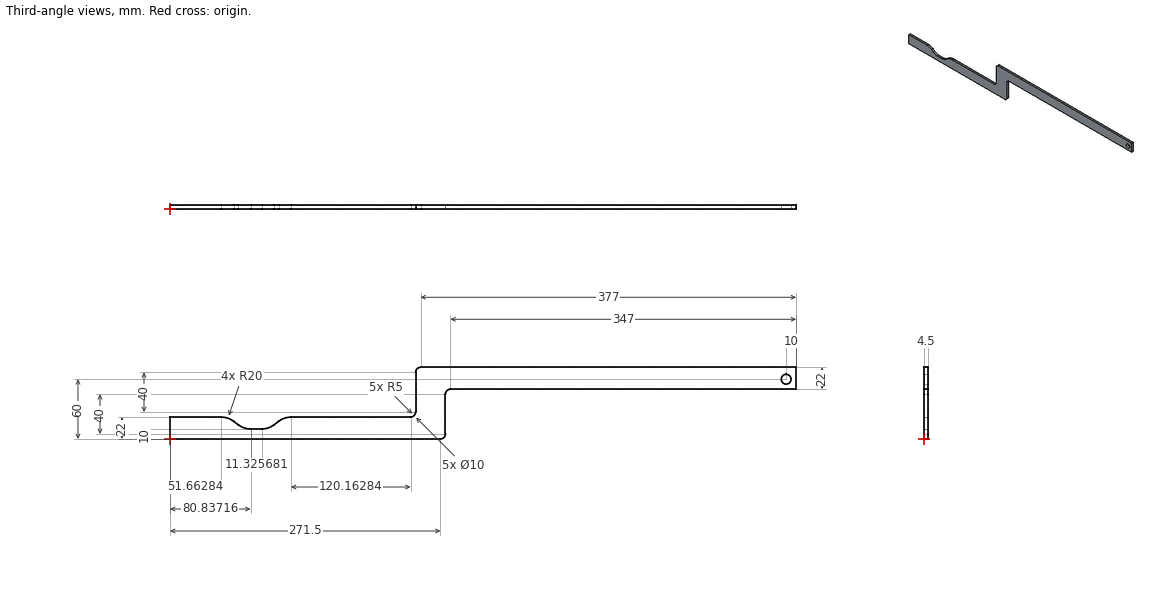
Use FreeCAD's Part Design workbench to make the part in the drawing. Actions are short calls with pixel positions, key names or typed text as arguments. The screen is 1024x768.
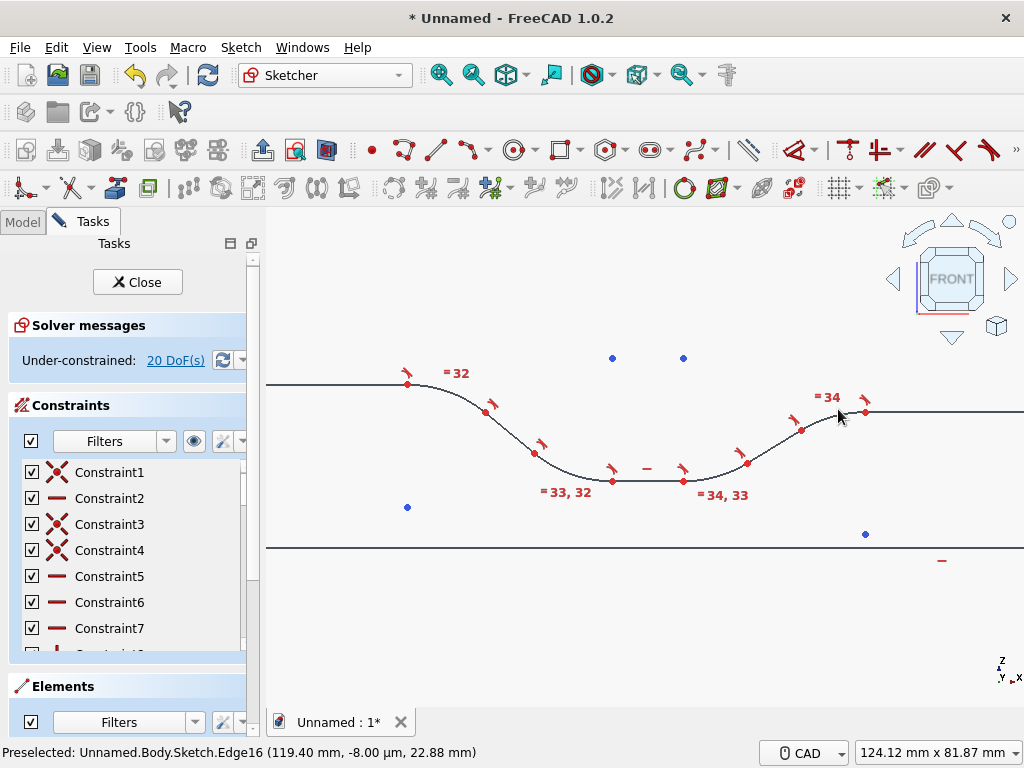
scroll(395, 473, down, 11)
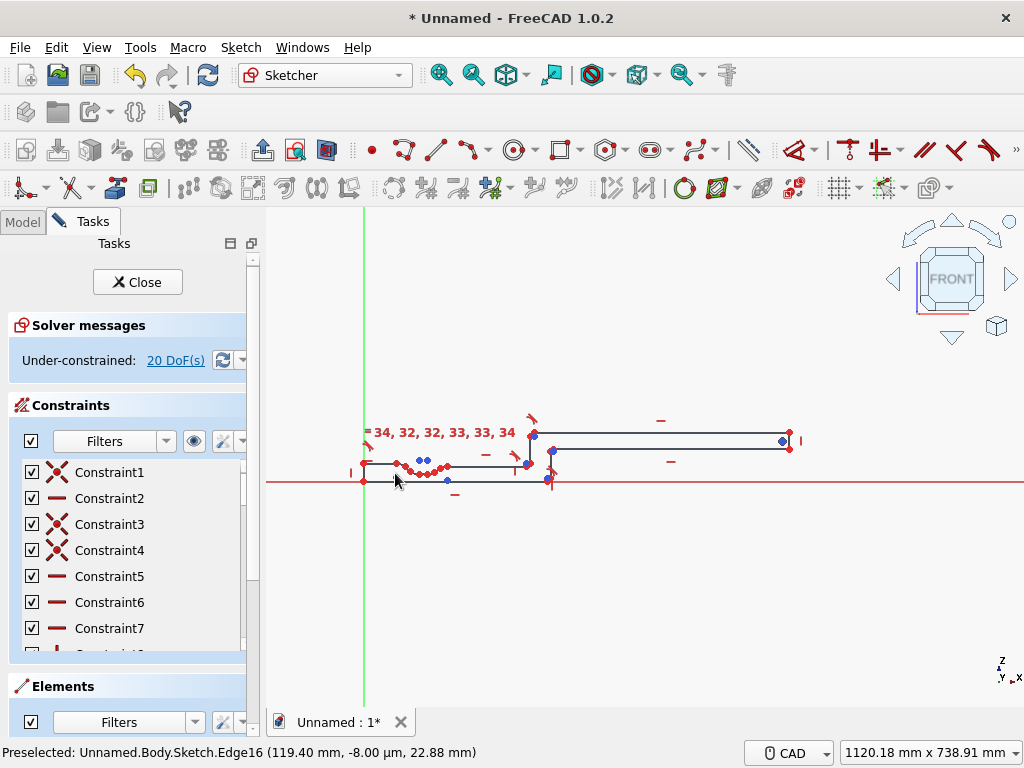
scroll(528, 466, up, 11)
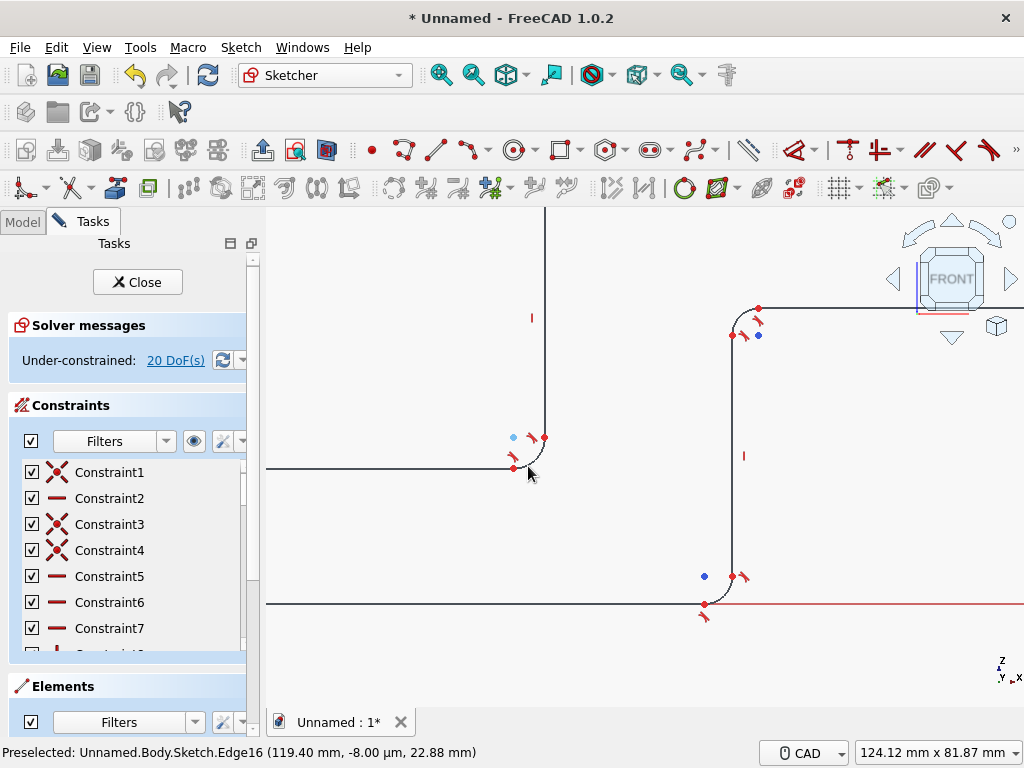
click(528, 465)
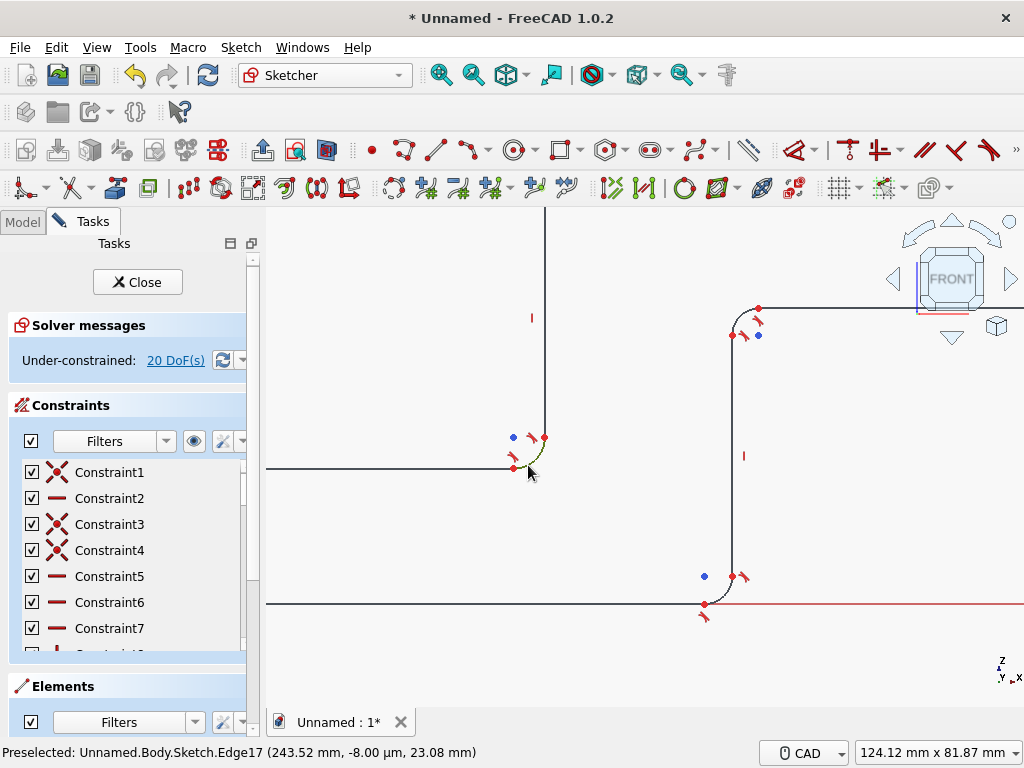
scroll(528, 466, down, 11)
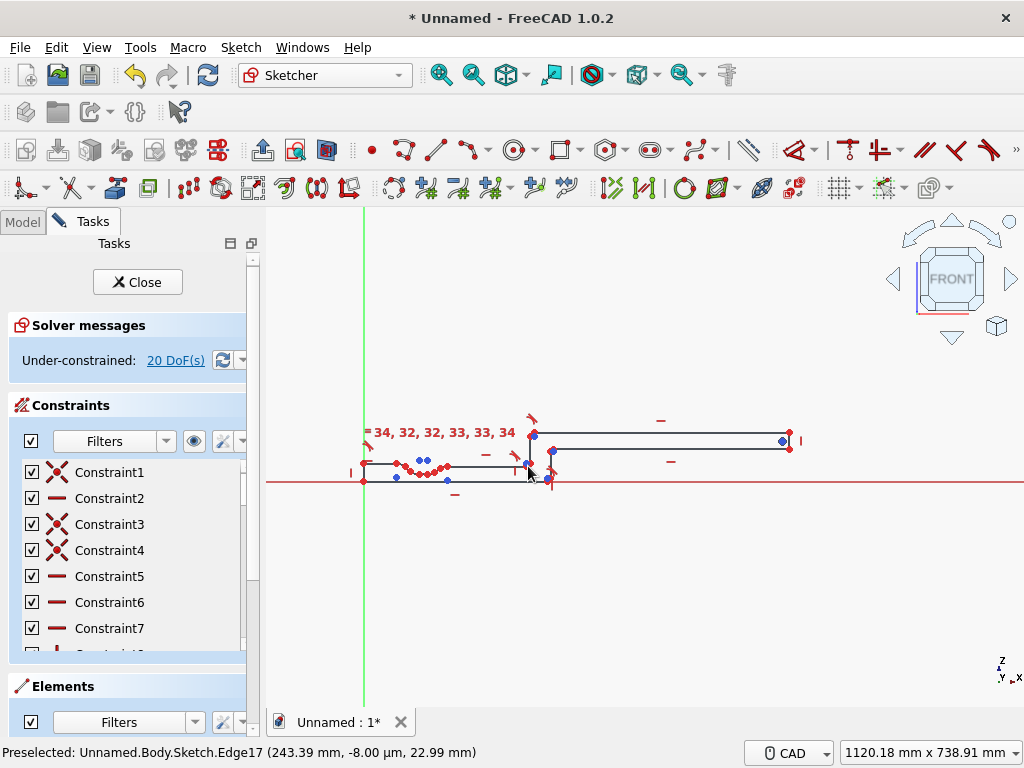
scroll(532, 433, up, 10)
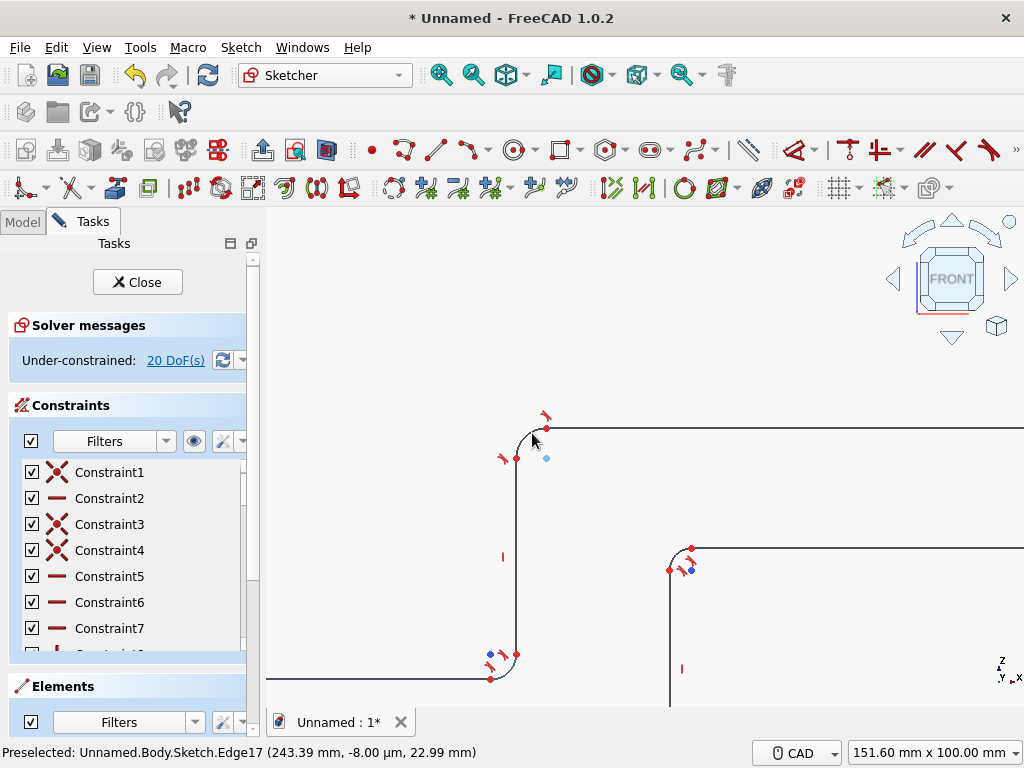
click(533, 432)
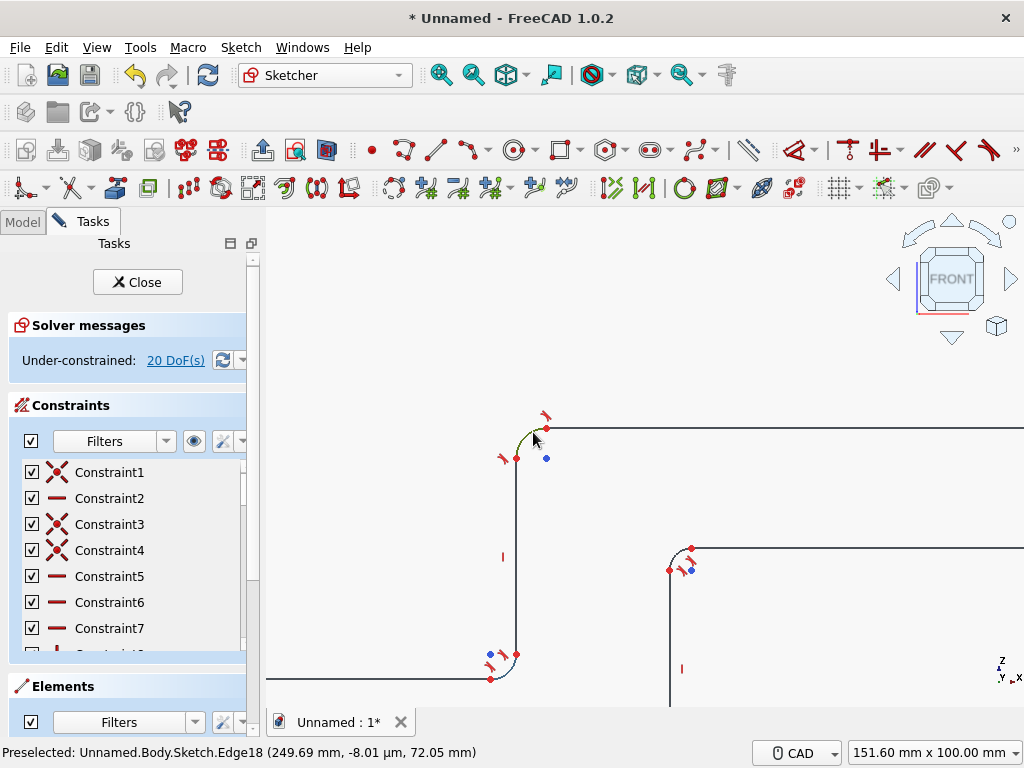
scroll(682, 551, up, 2)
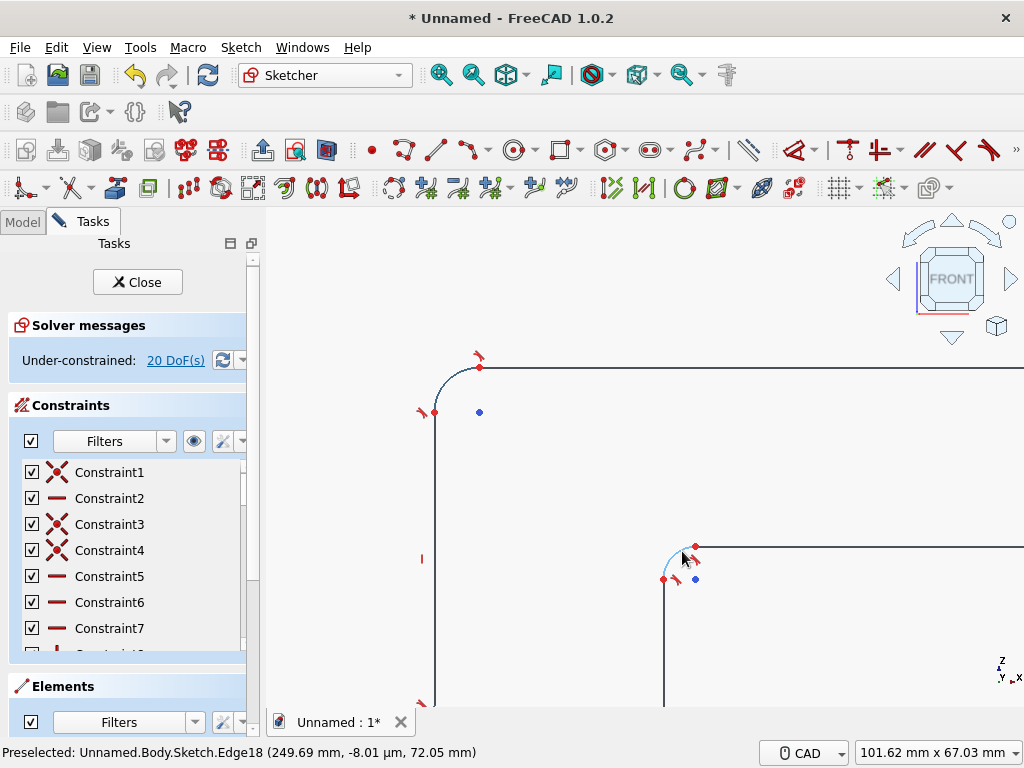
click(681, 550)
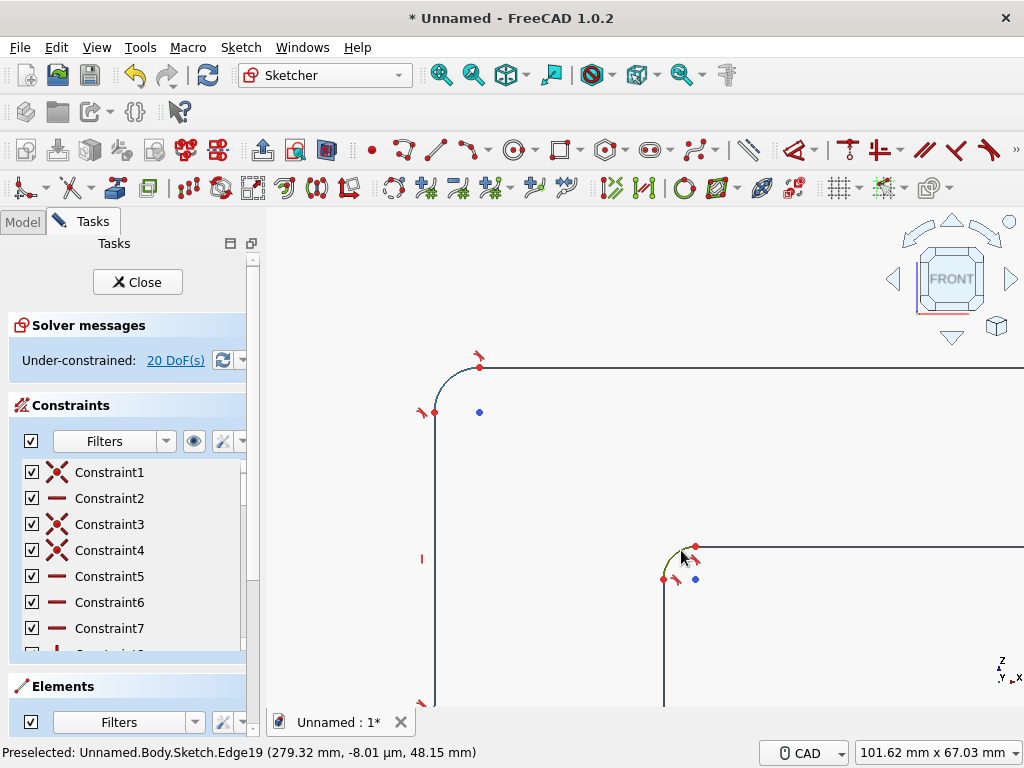
scroll(540, 439, down, 12)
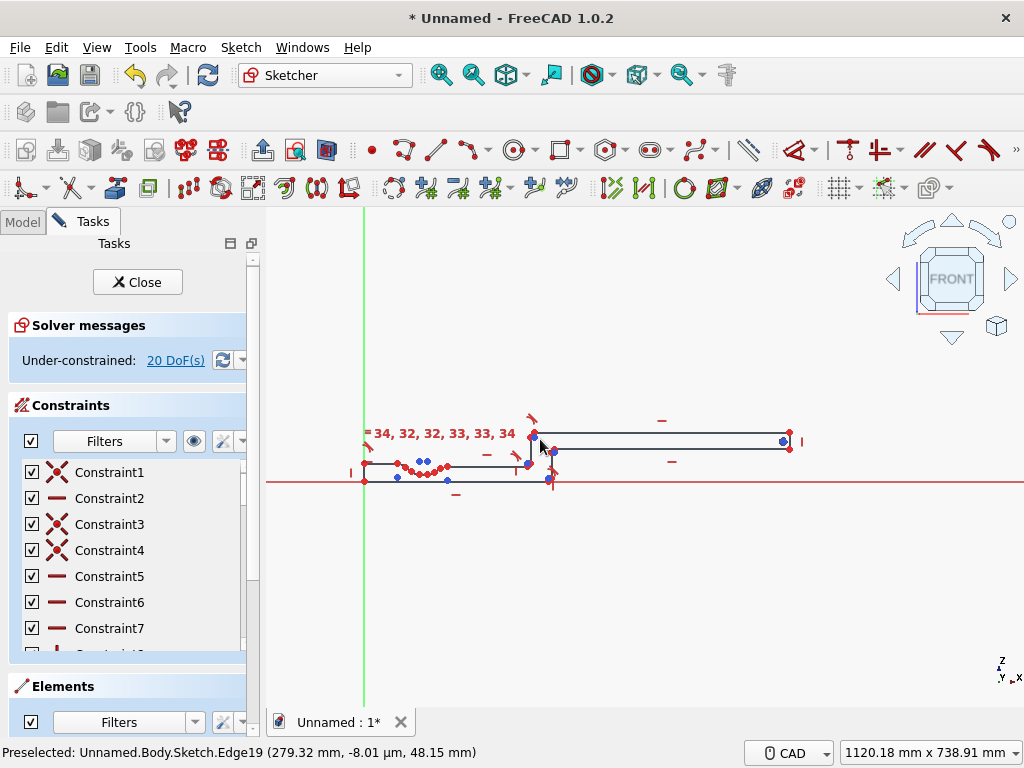
scroll(550, 482, up, 12)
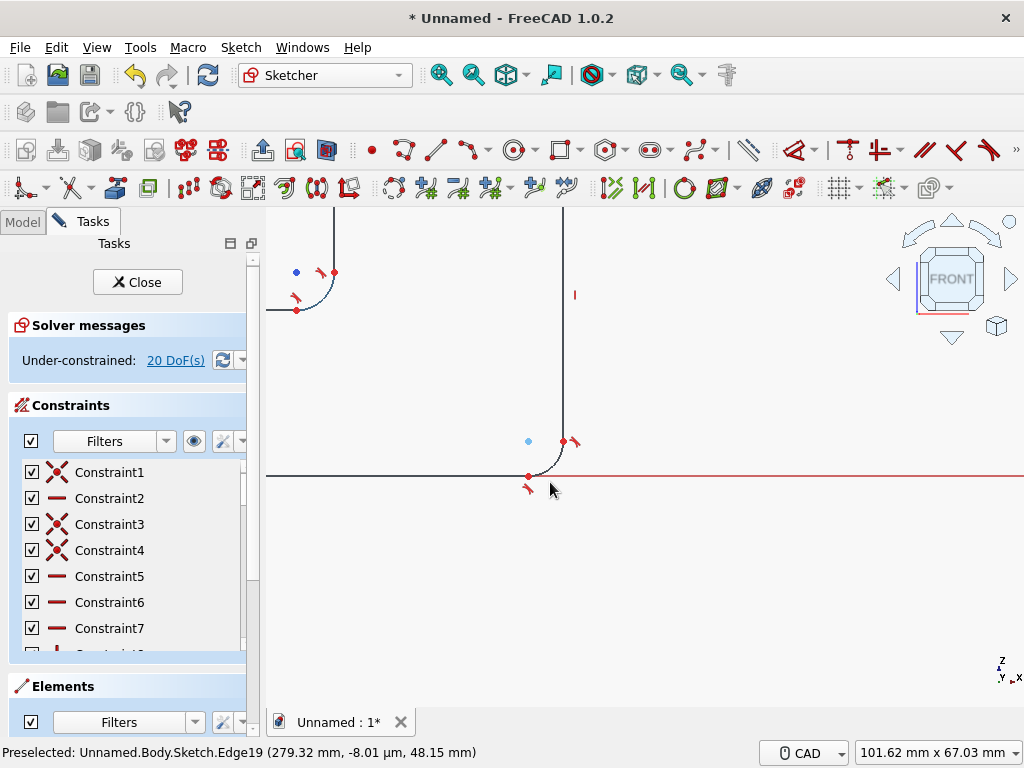
click(544, 472)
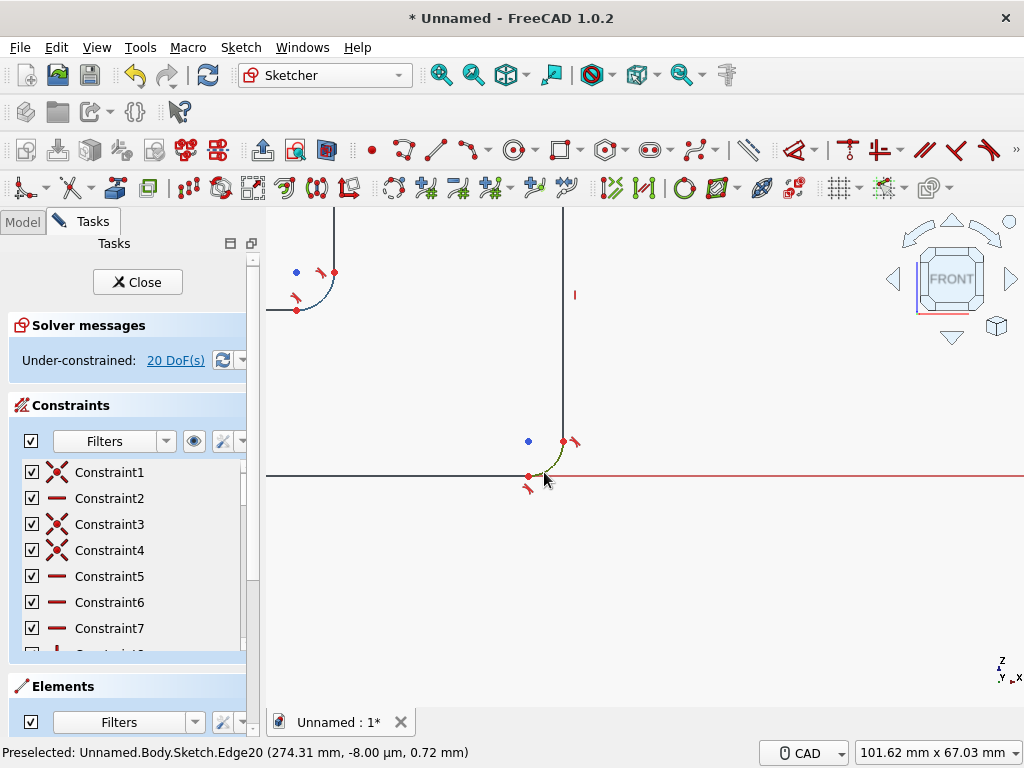
key(e)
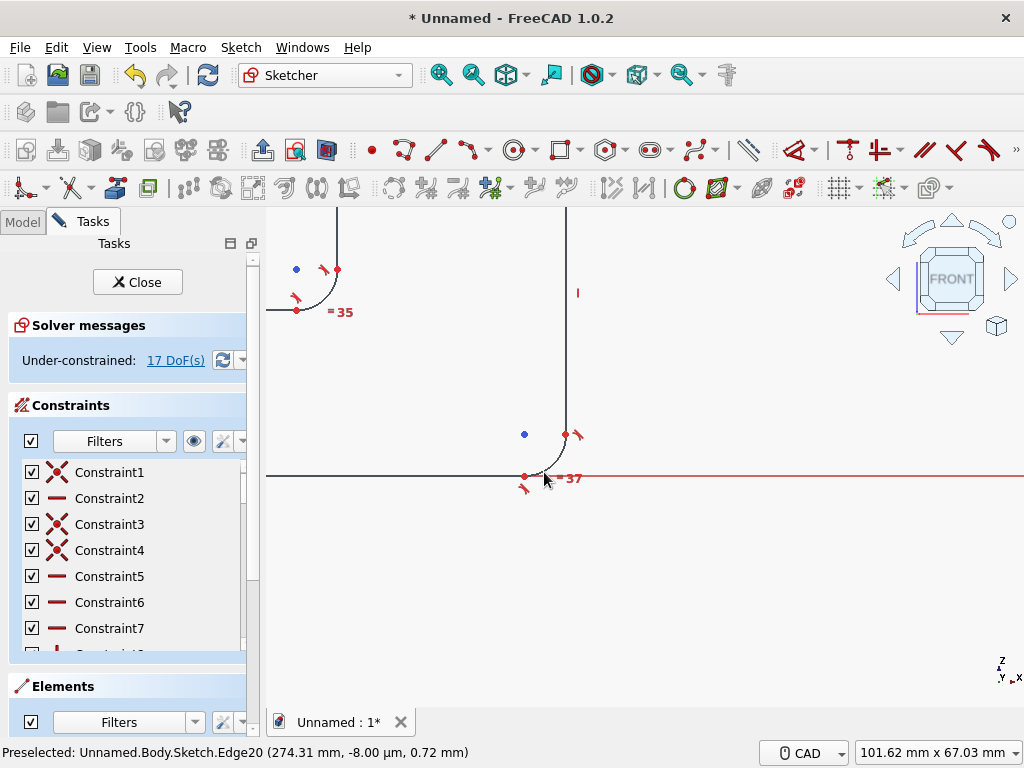
key(d)